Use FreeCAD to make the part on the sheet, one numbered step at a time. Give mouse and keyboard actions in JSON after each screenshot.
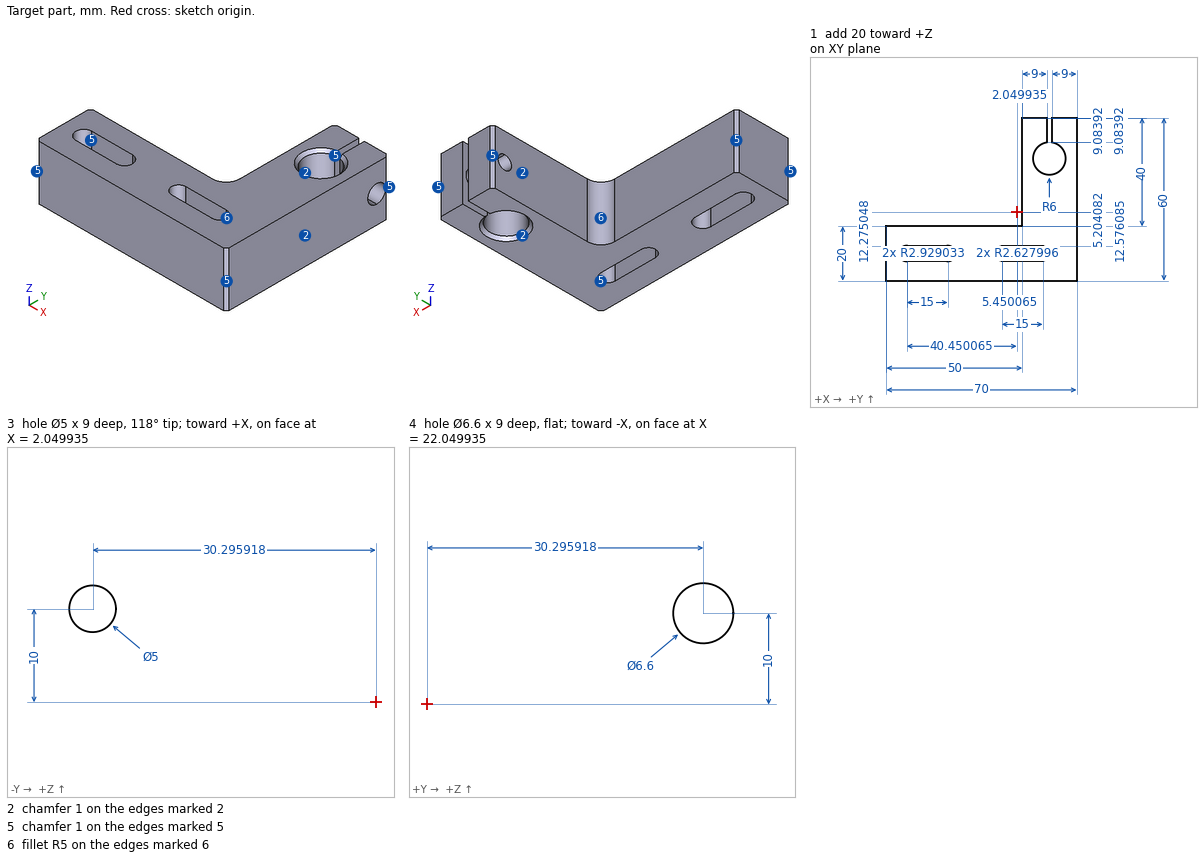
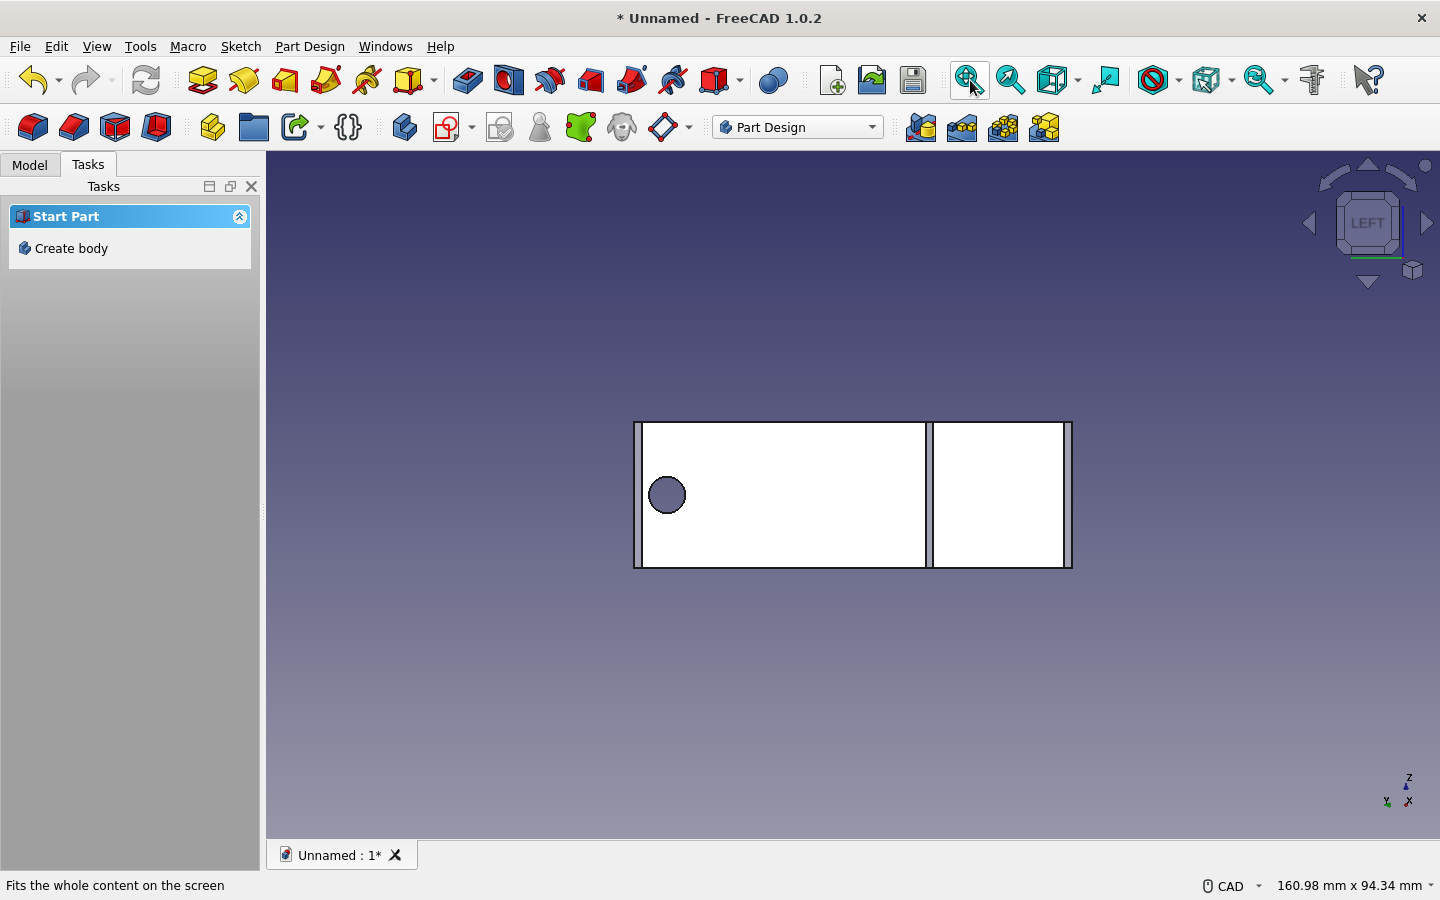
{"action": "left_click", "coordinate": [970, 80]}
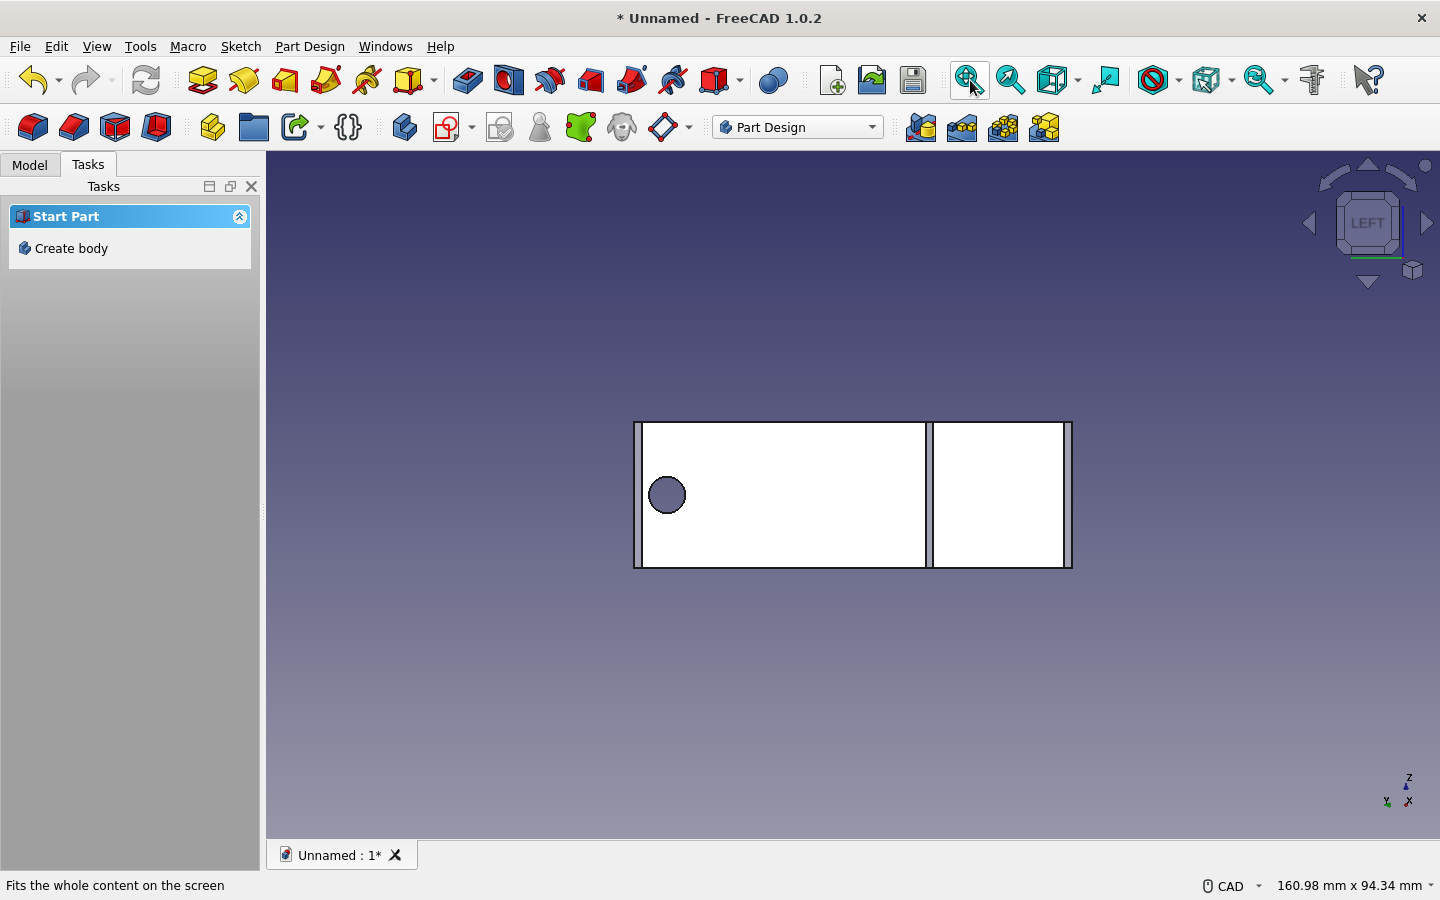
{"action": "key", "text": "v 3"}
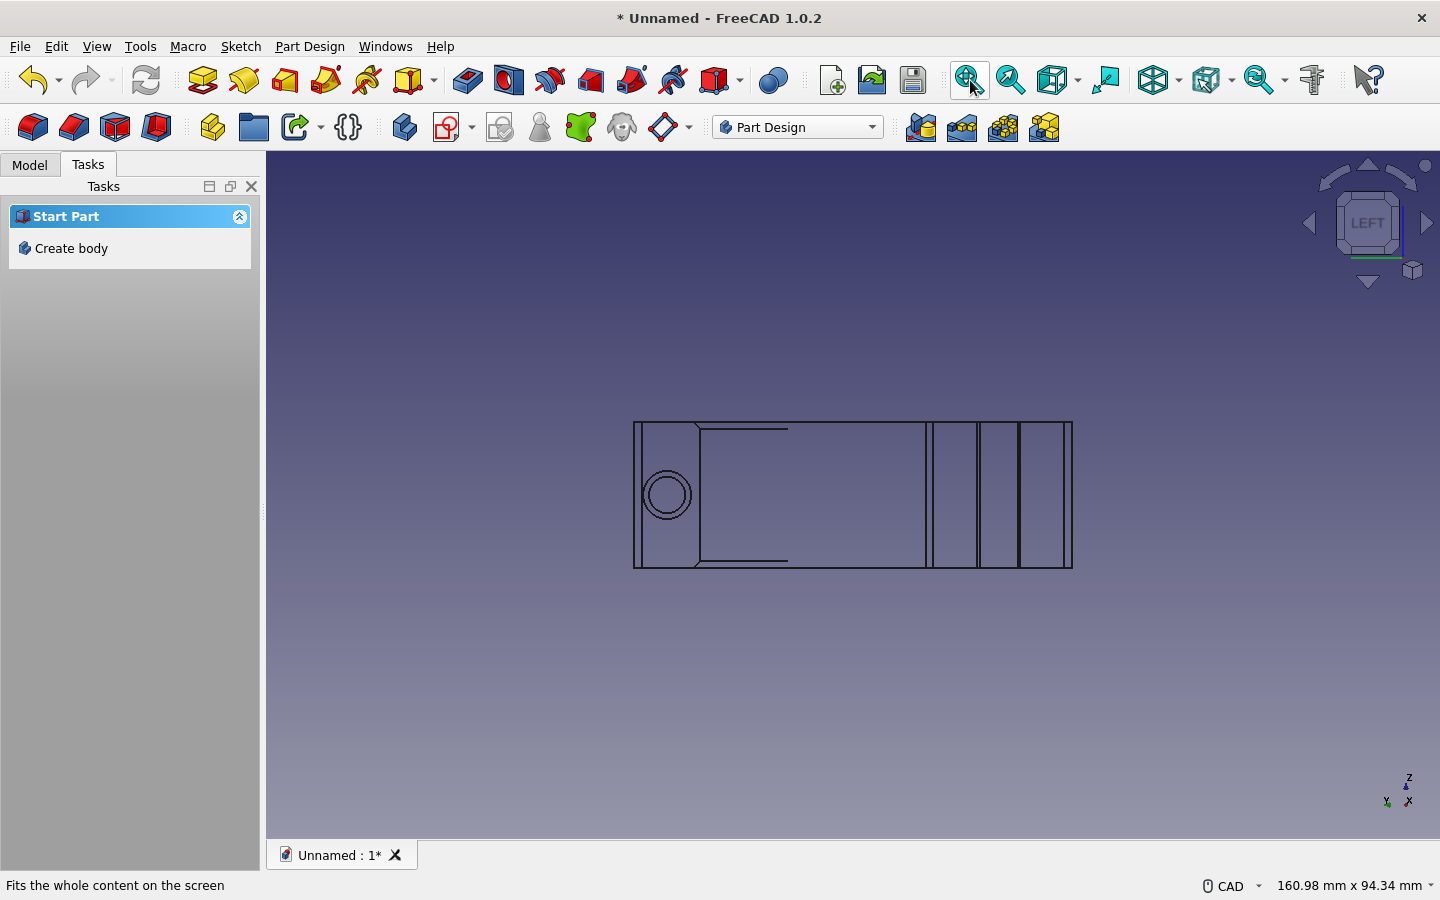
{"action": "key", "text": "0"}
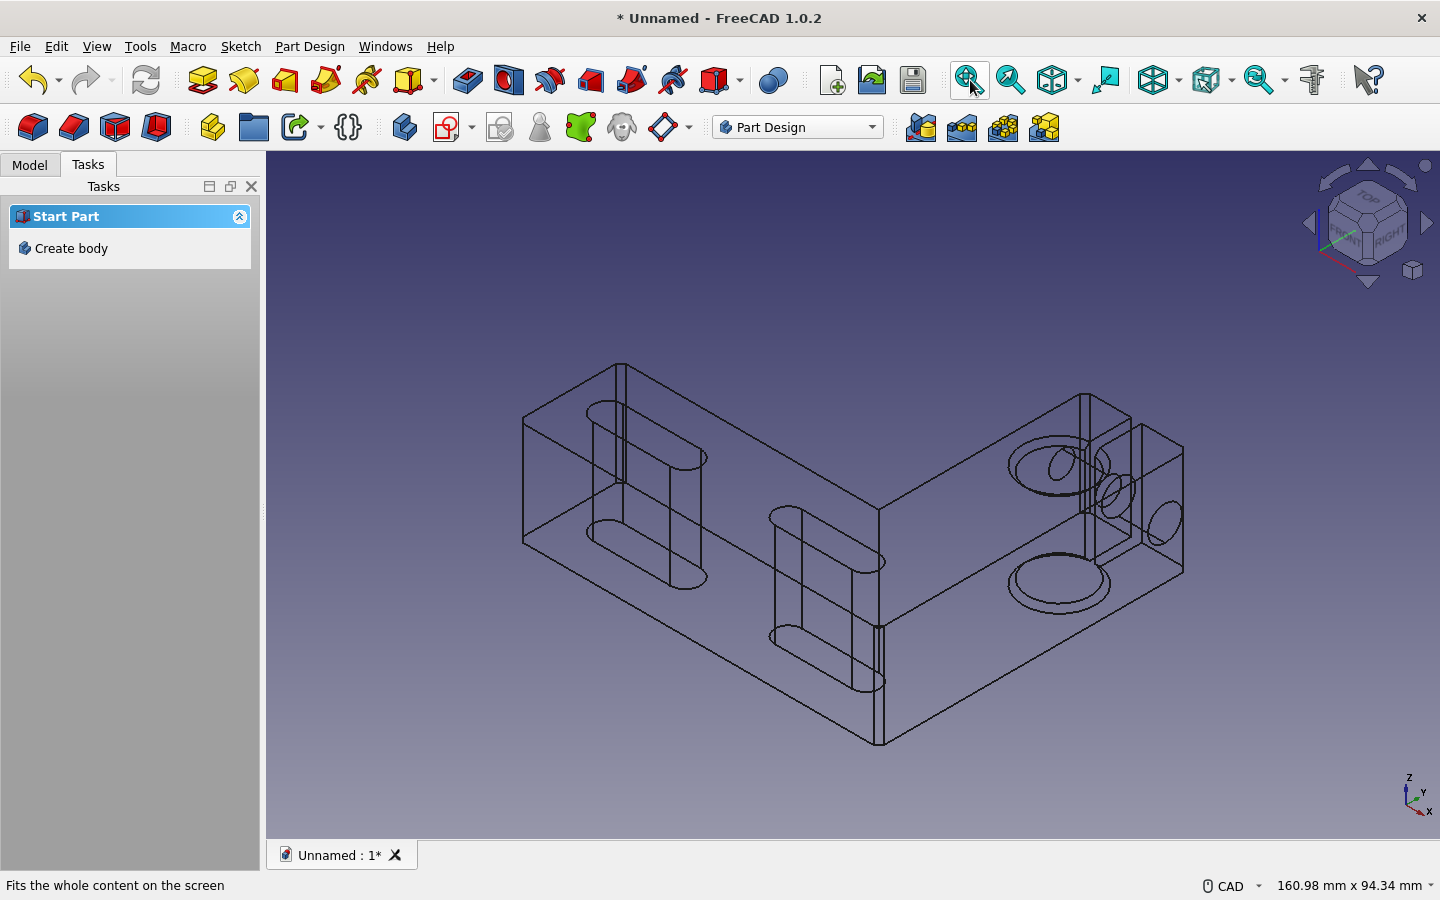
{"action": "left_click", "coordinate": [879, 545]}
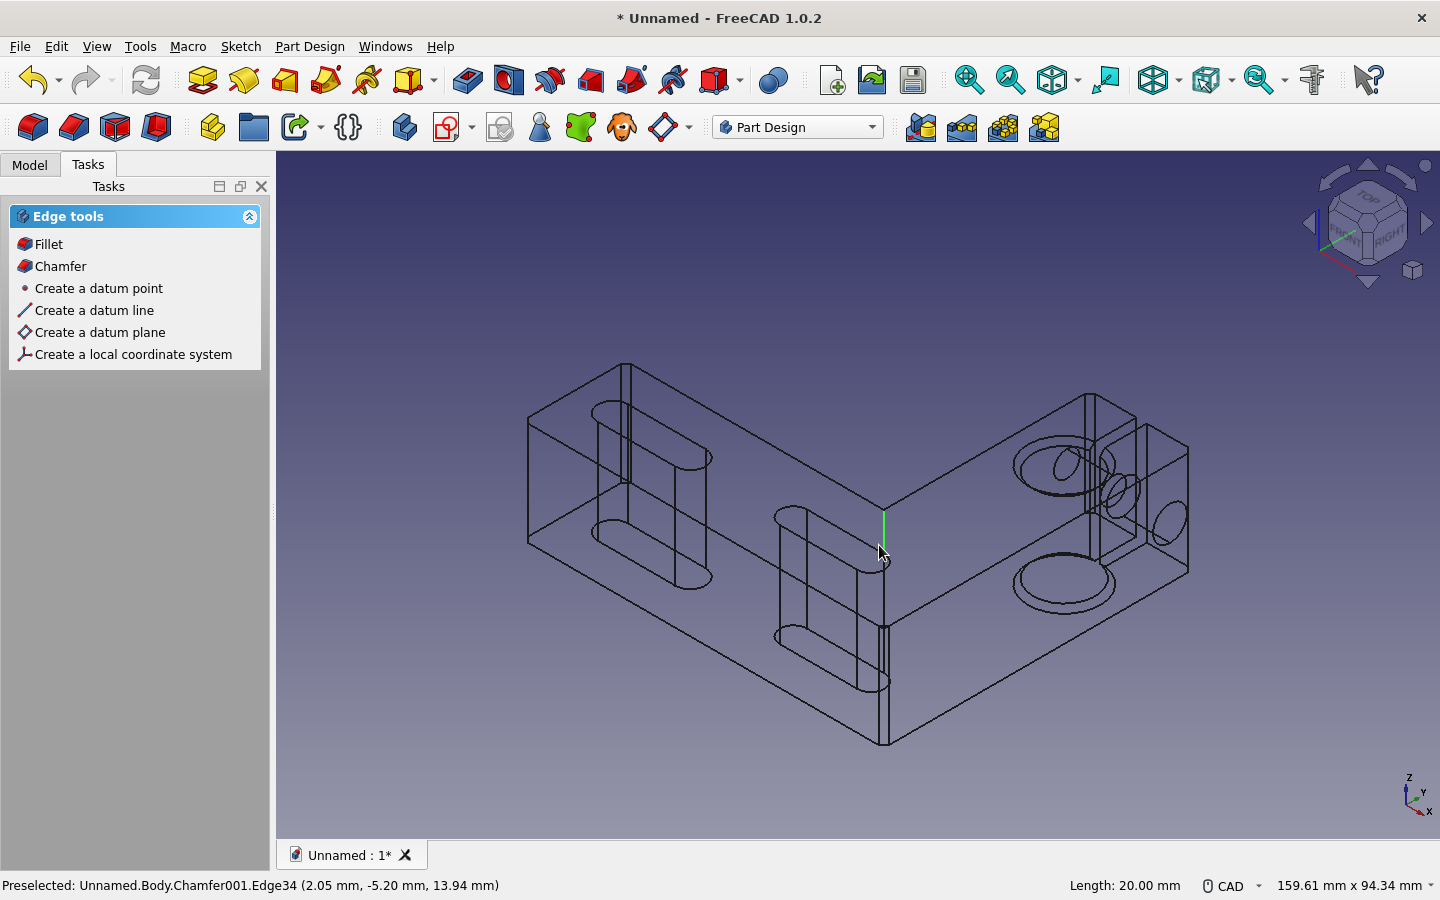
{"action": "key", "text": "v 1"}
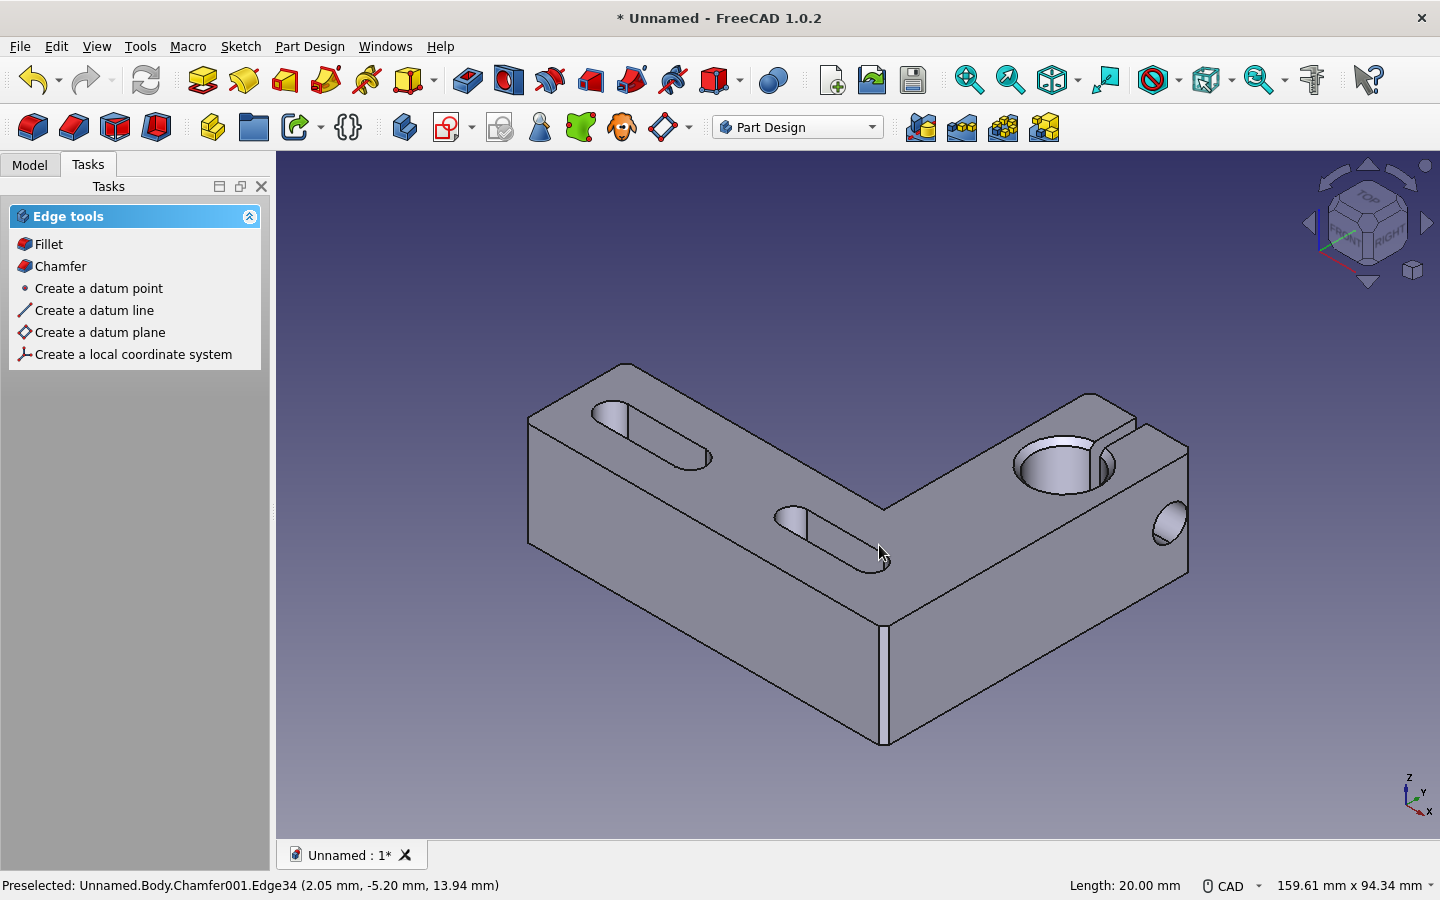
{"action": "left_click", "coordinate": [33, 128]}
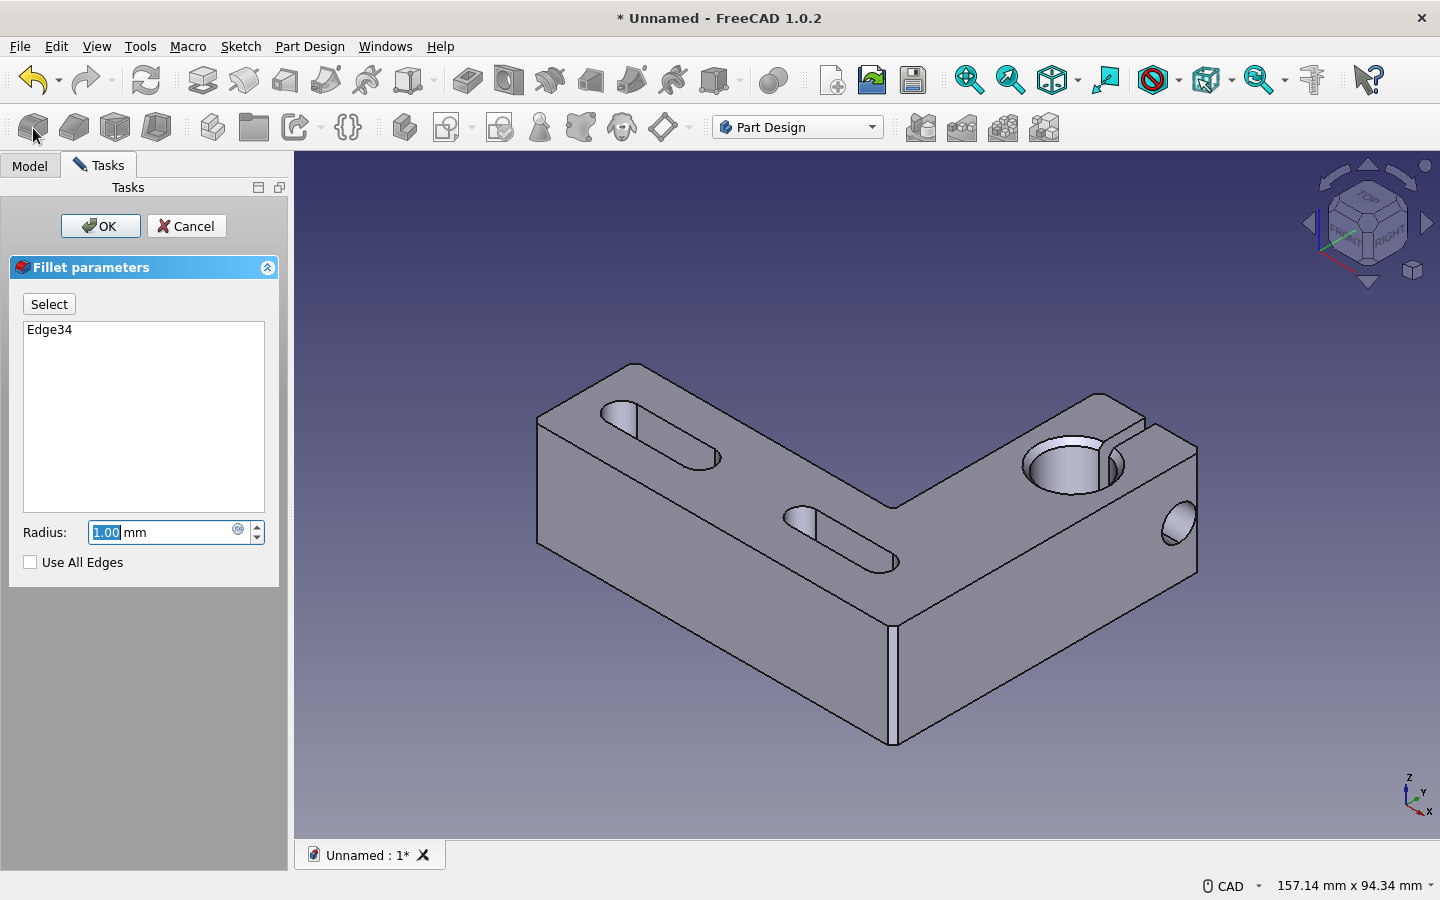
{"action": "type", "text": "5"}
{"action": "key", "text": "Tab"}